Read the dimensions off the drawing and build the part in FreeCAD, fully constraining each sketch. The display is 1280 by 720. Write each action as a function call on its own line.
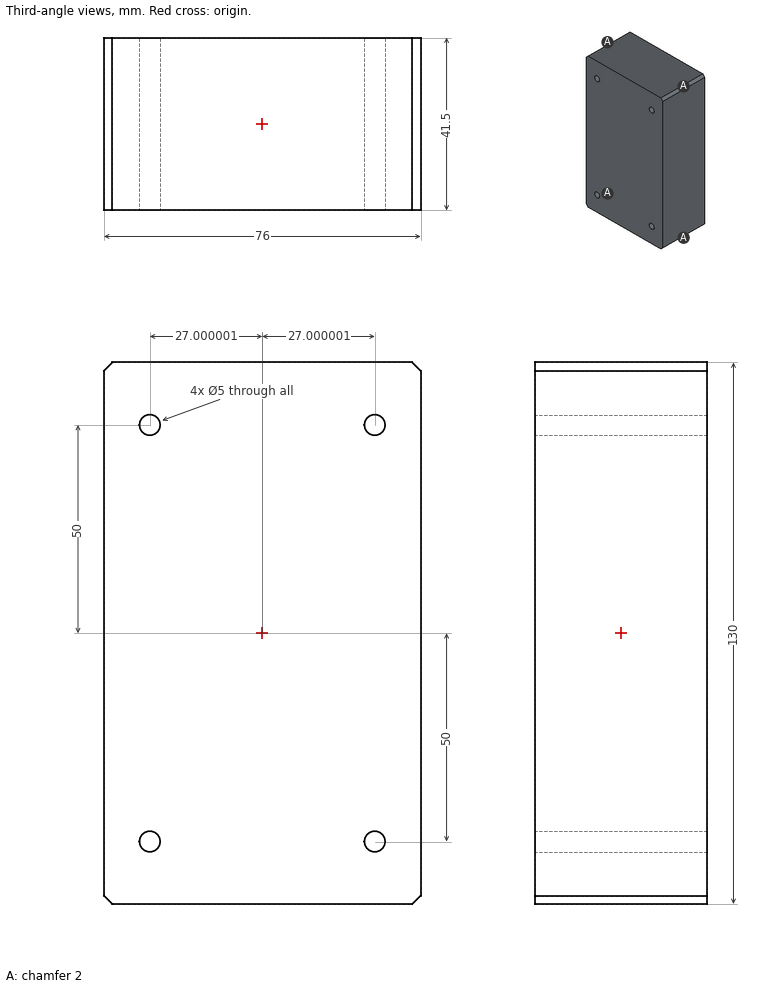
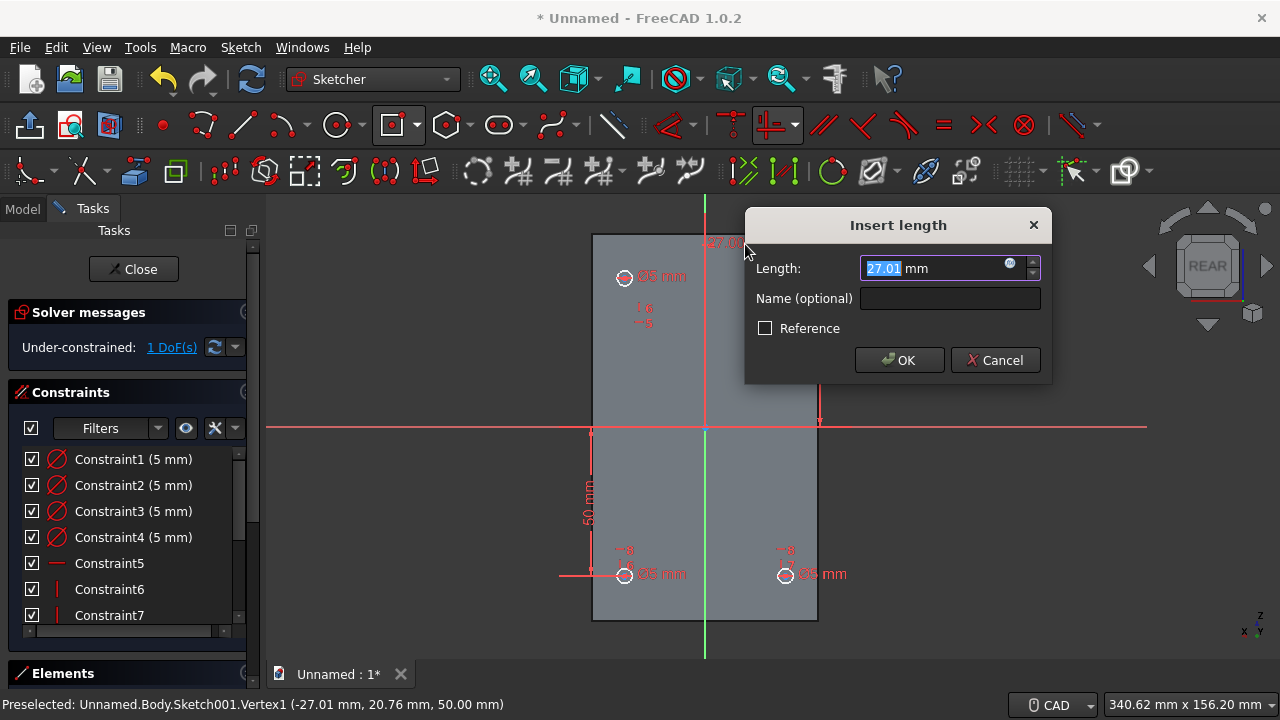
text(27.000001)
key(Return)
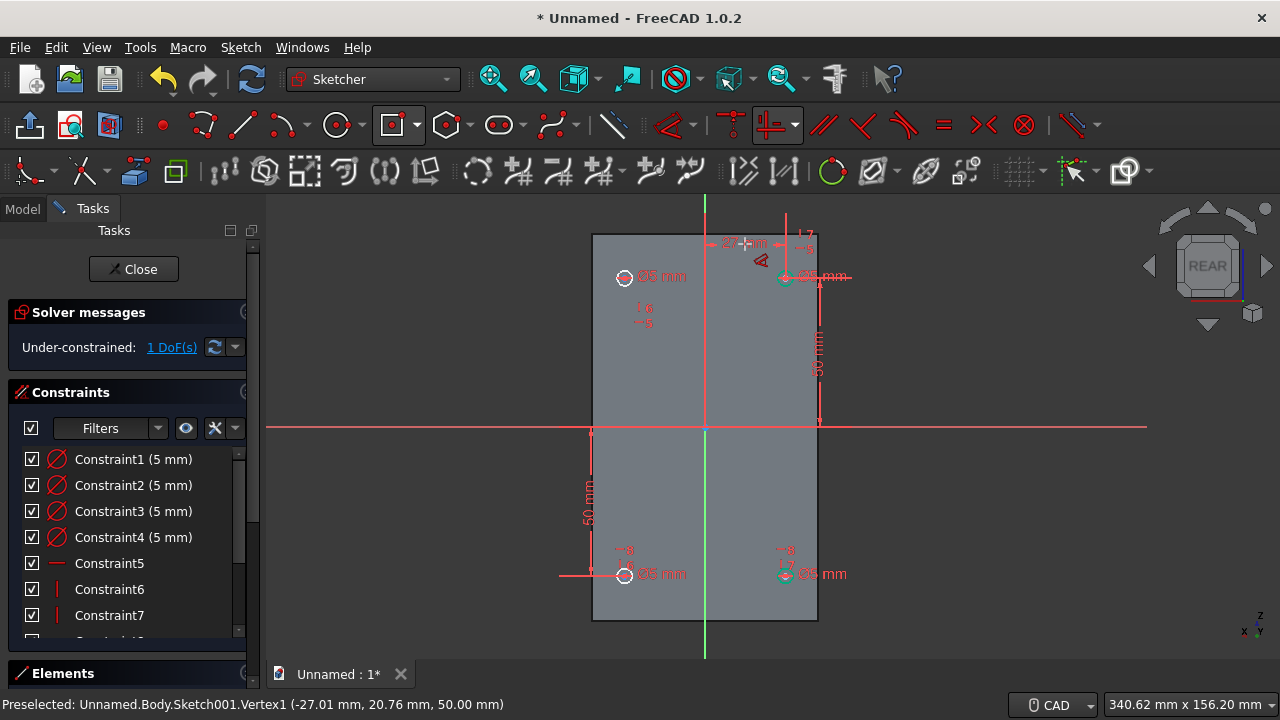
click(625, 278)
click(665, 244)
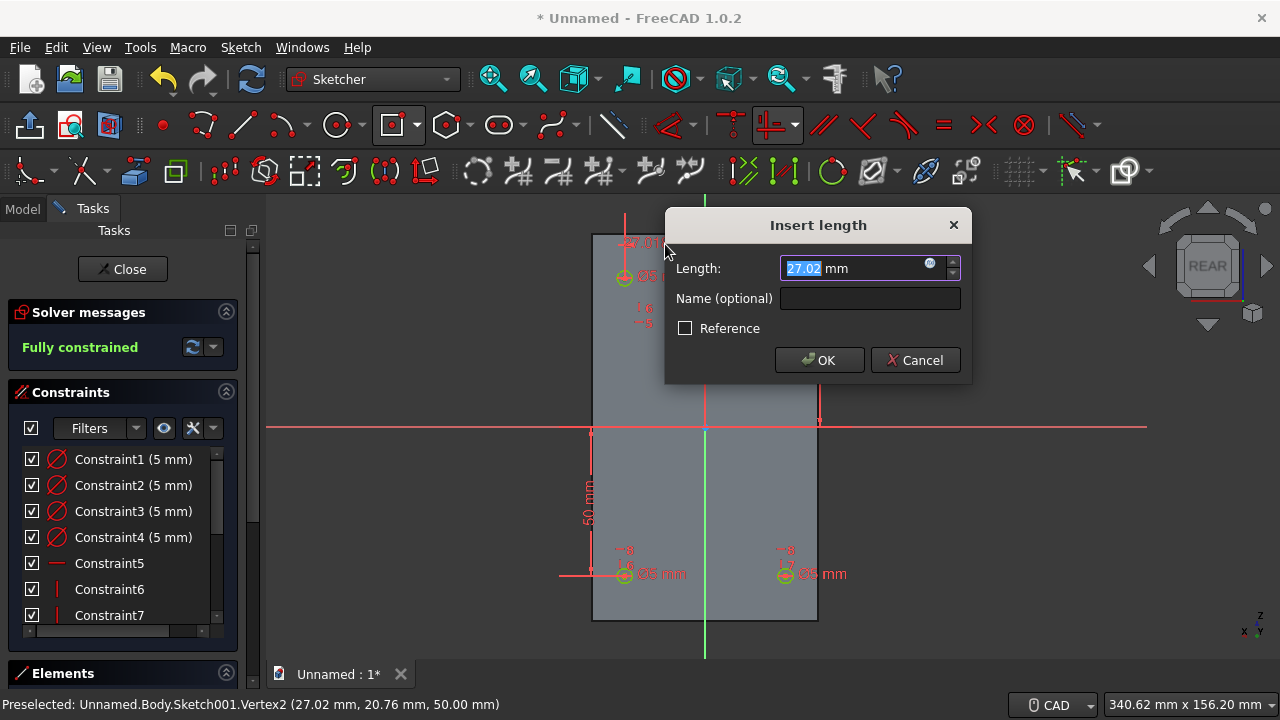
text(27.000001)
key(Return)
key(Escape)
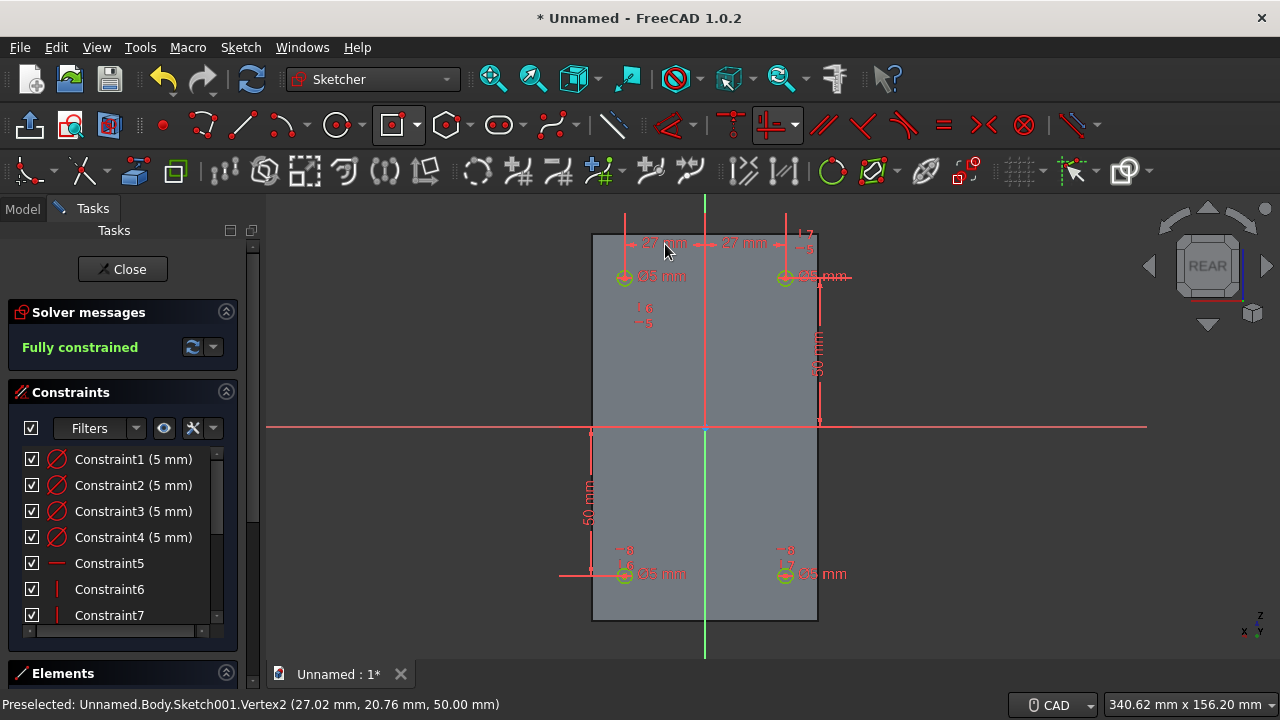
click(123, 269)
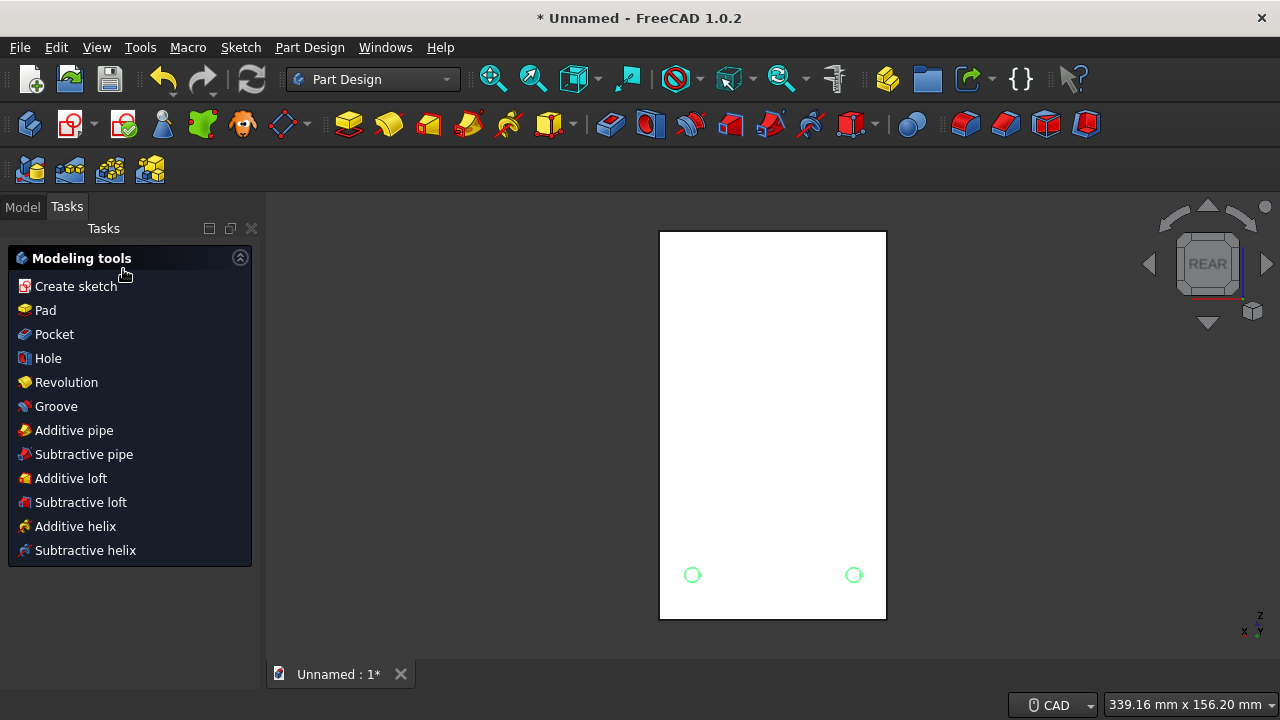
click(652, 124)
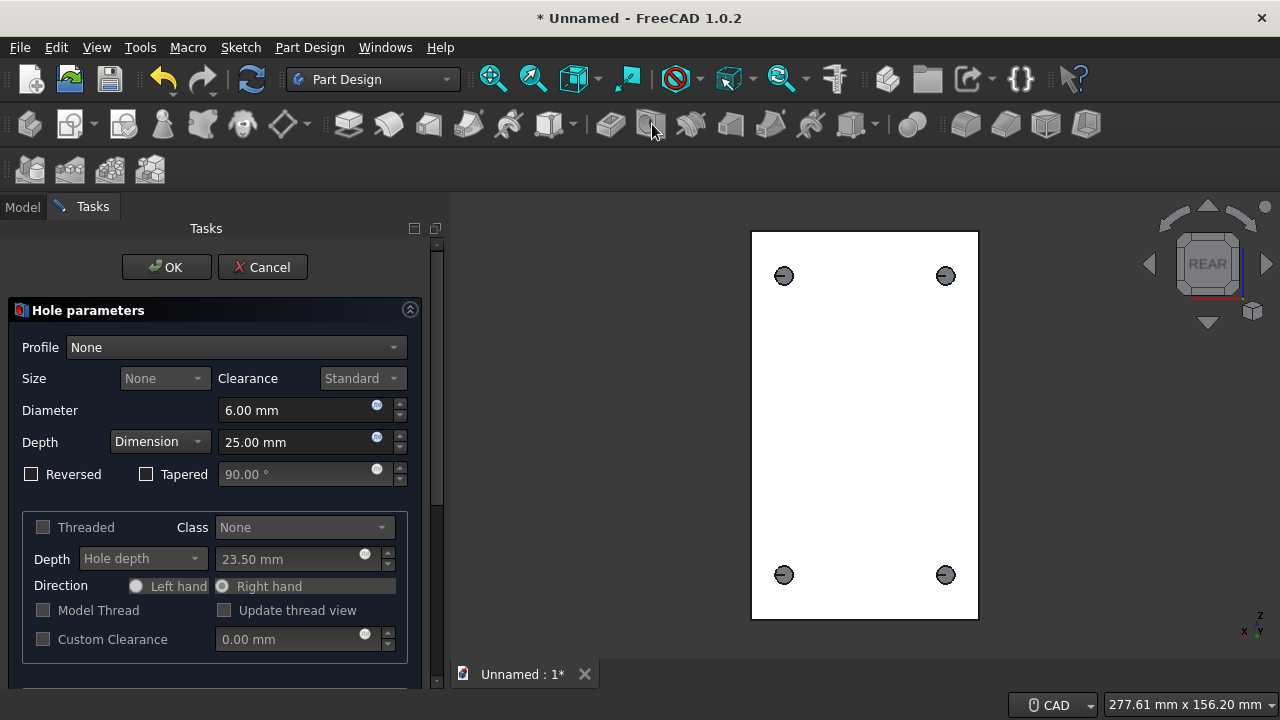
triple_click(305, 410)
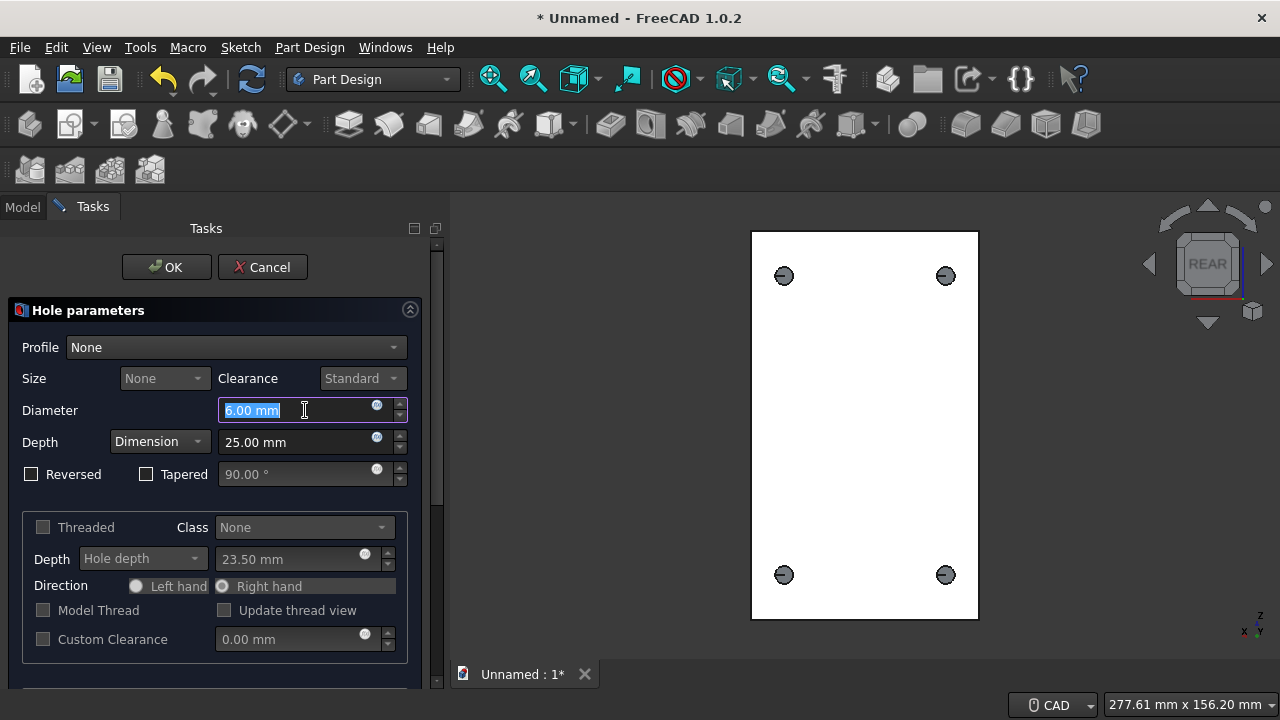
text(5)
key(Tab)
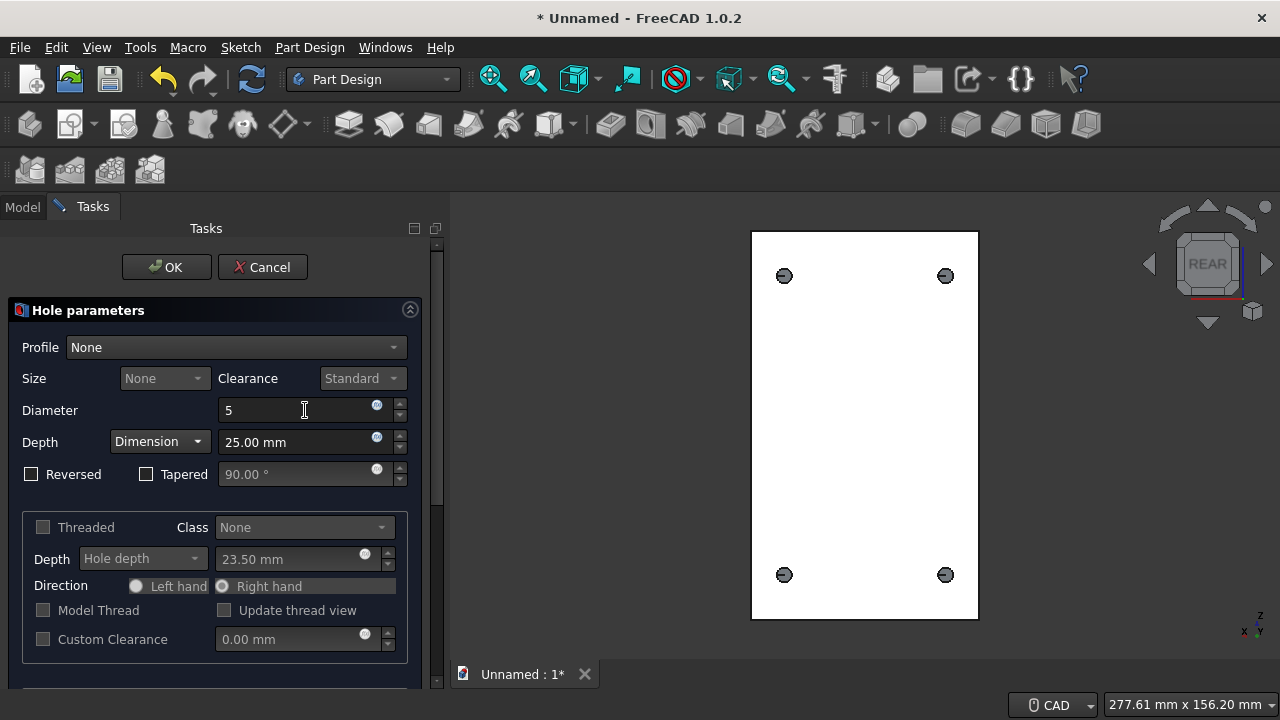
click(161, 442)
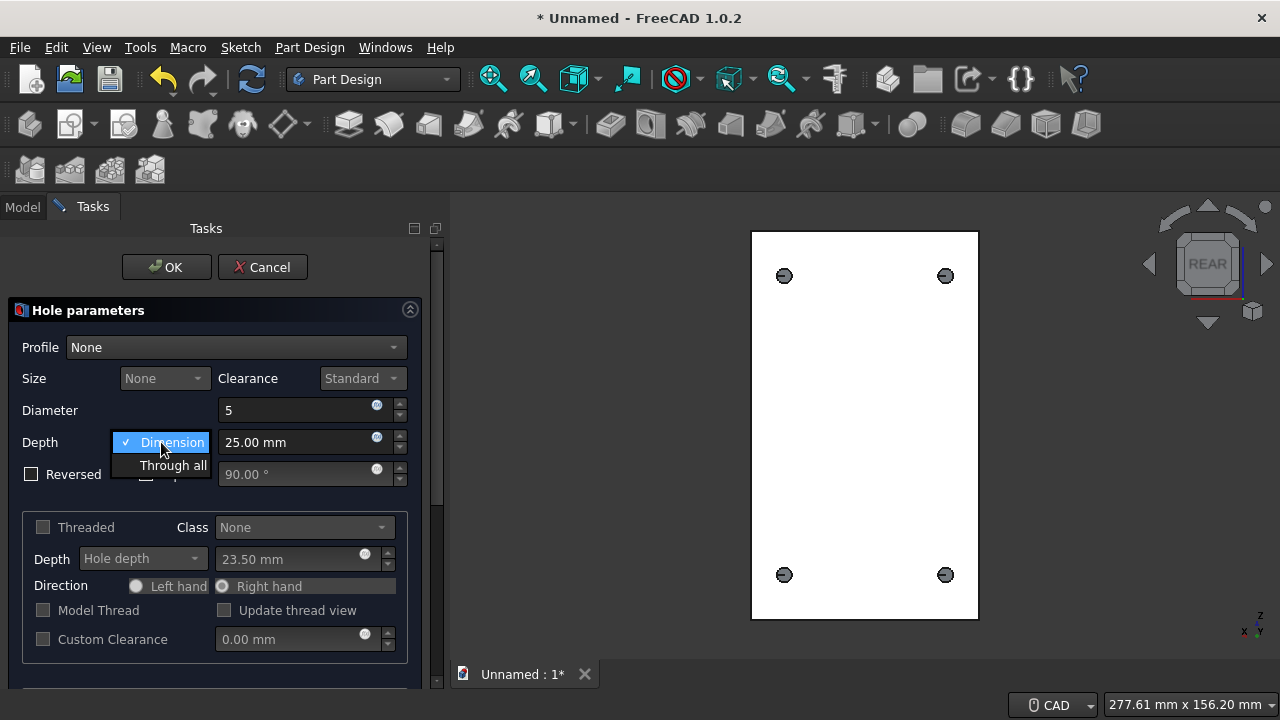
click(160, 466)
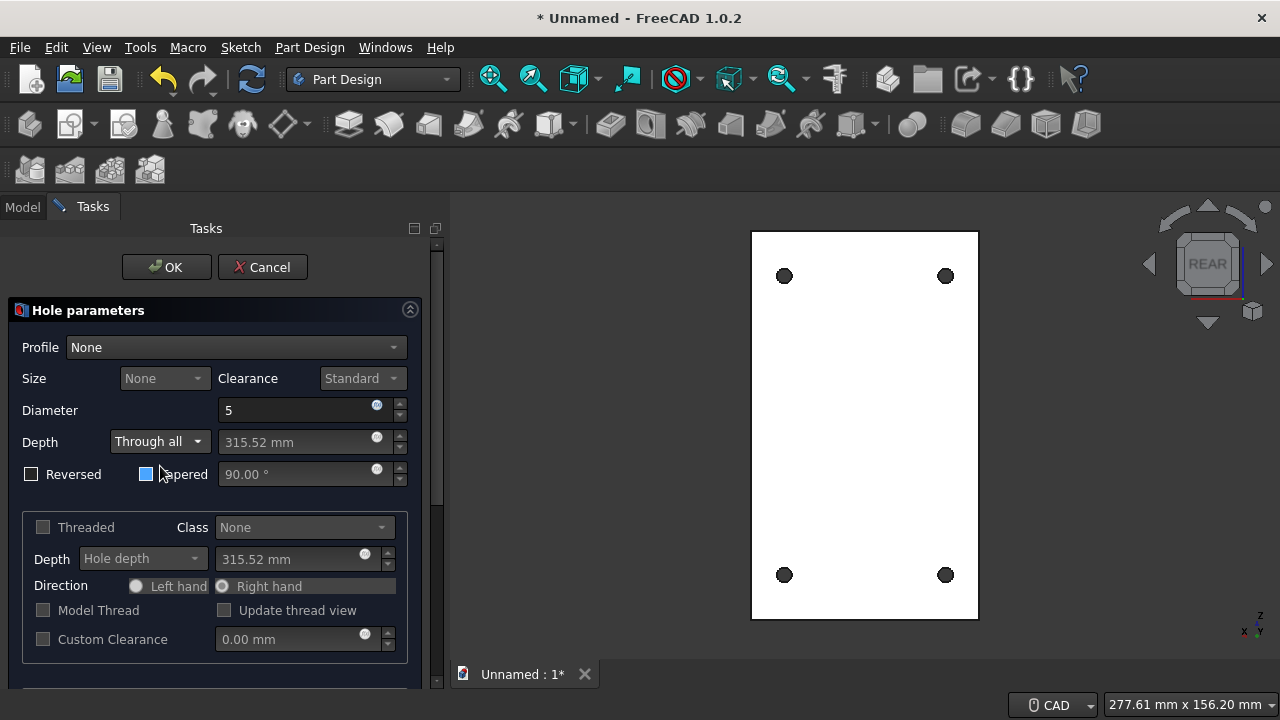
click(167, 267)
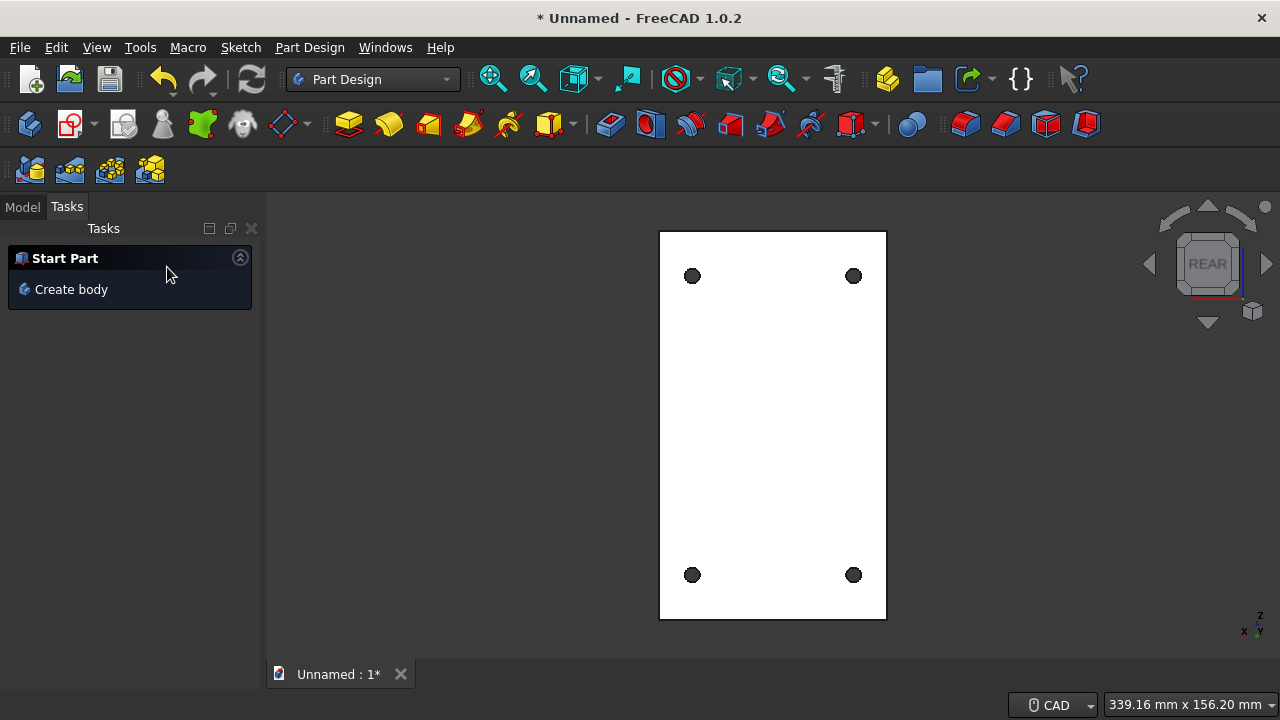
key(0)